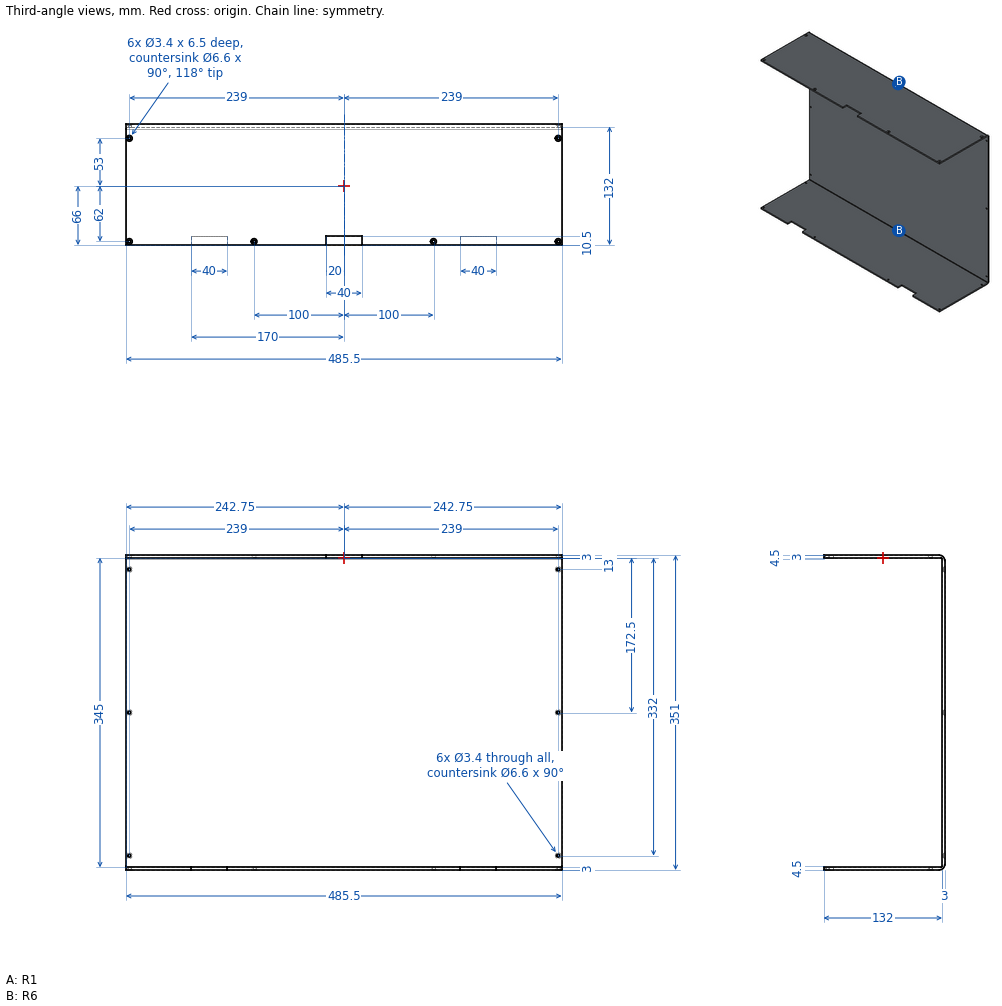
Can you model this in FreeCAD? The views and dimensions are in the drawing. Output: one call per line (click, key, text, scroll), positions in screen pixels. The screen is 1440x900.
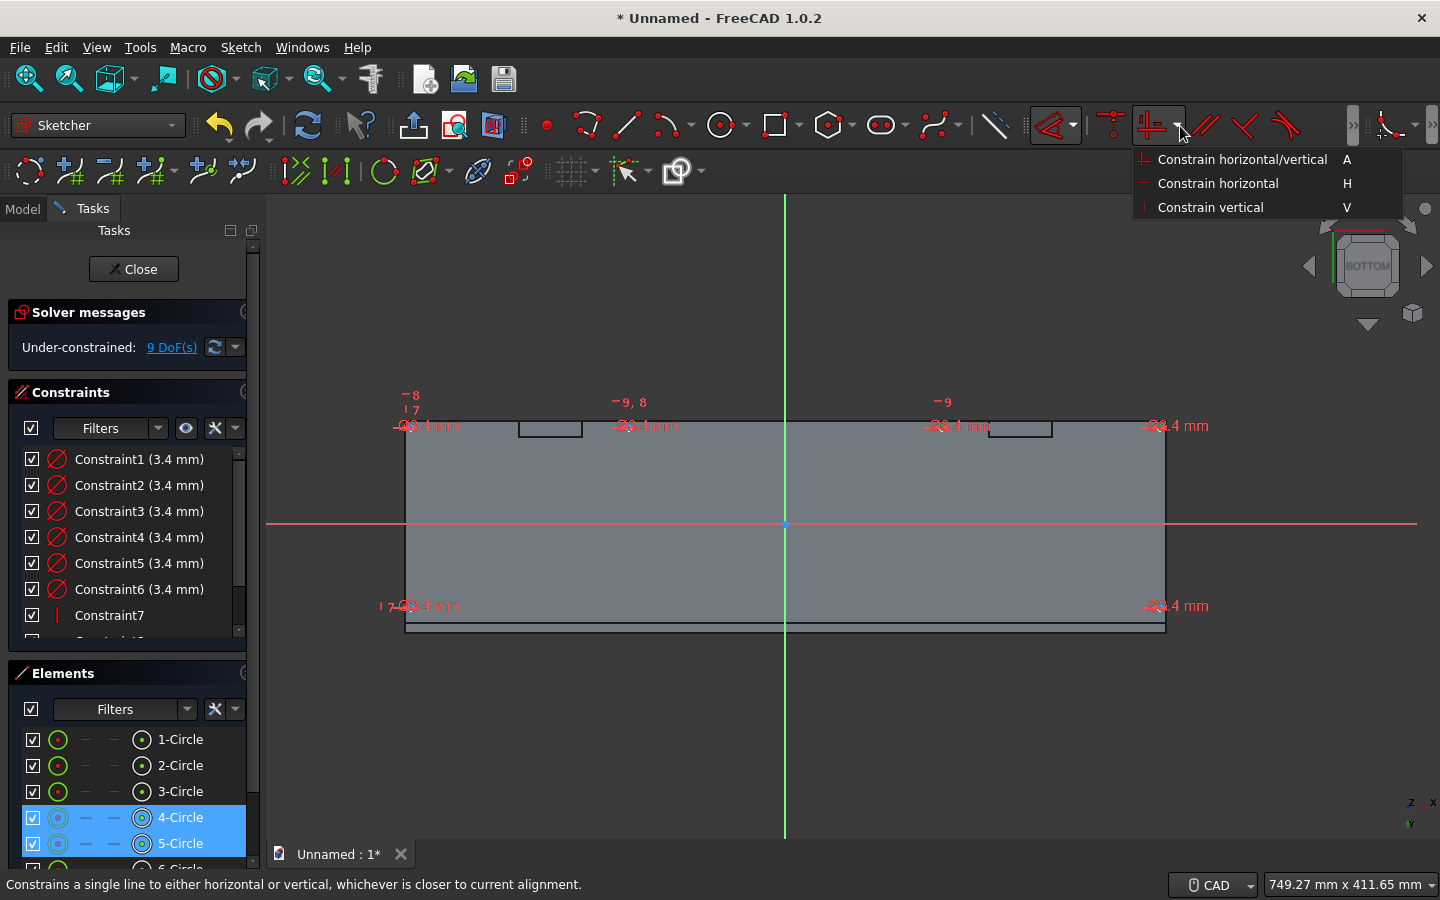
click(1268, 183)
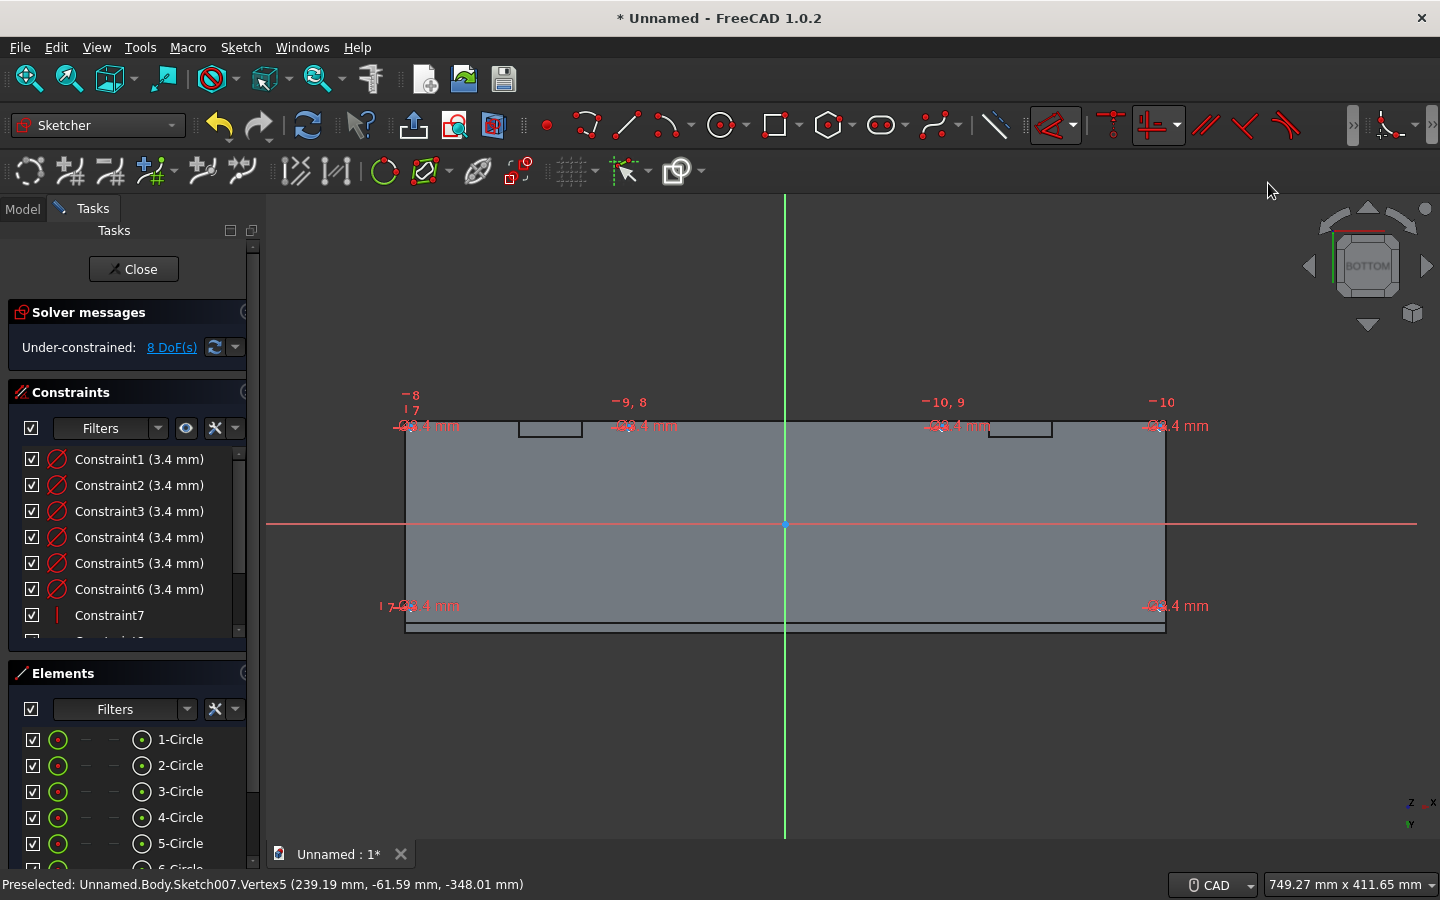
click(1160, 428)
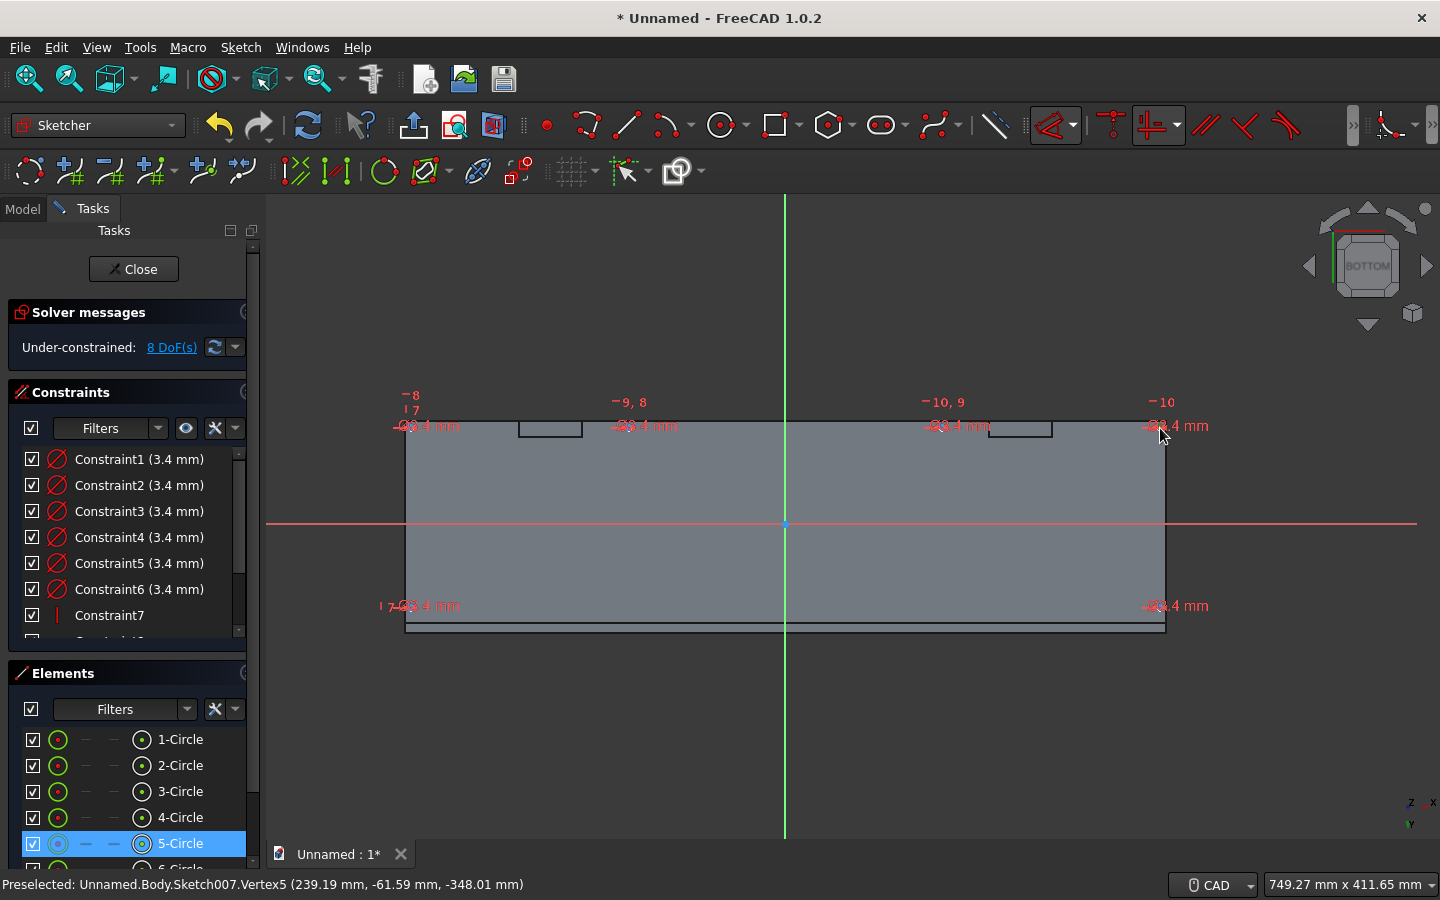
click(1160, 608)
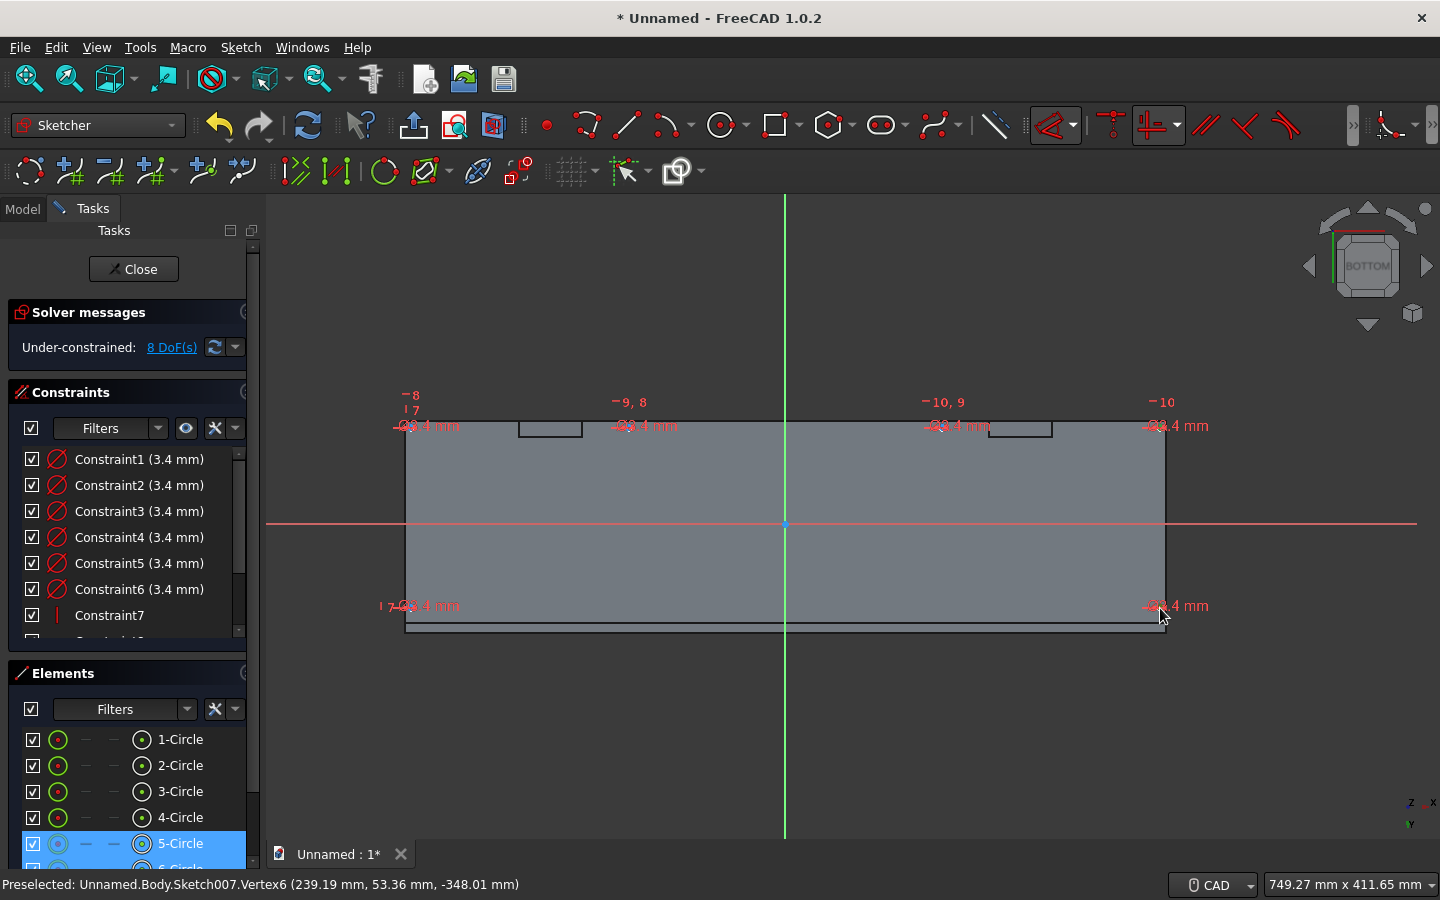
click(1180, 126)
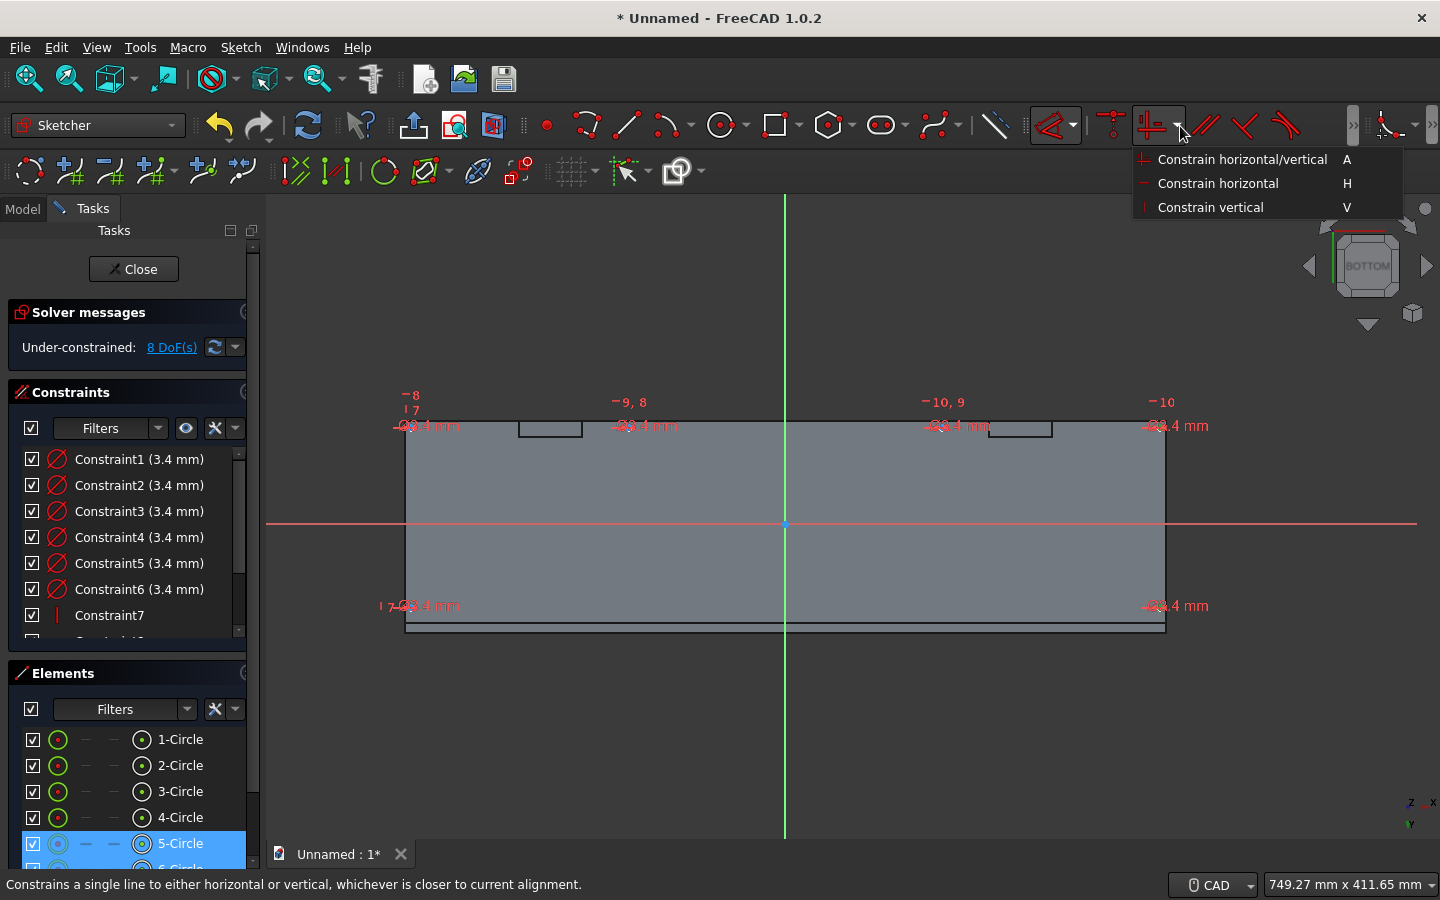
click(1268, 207)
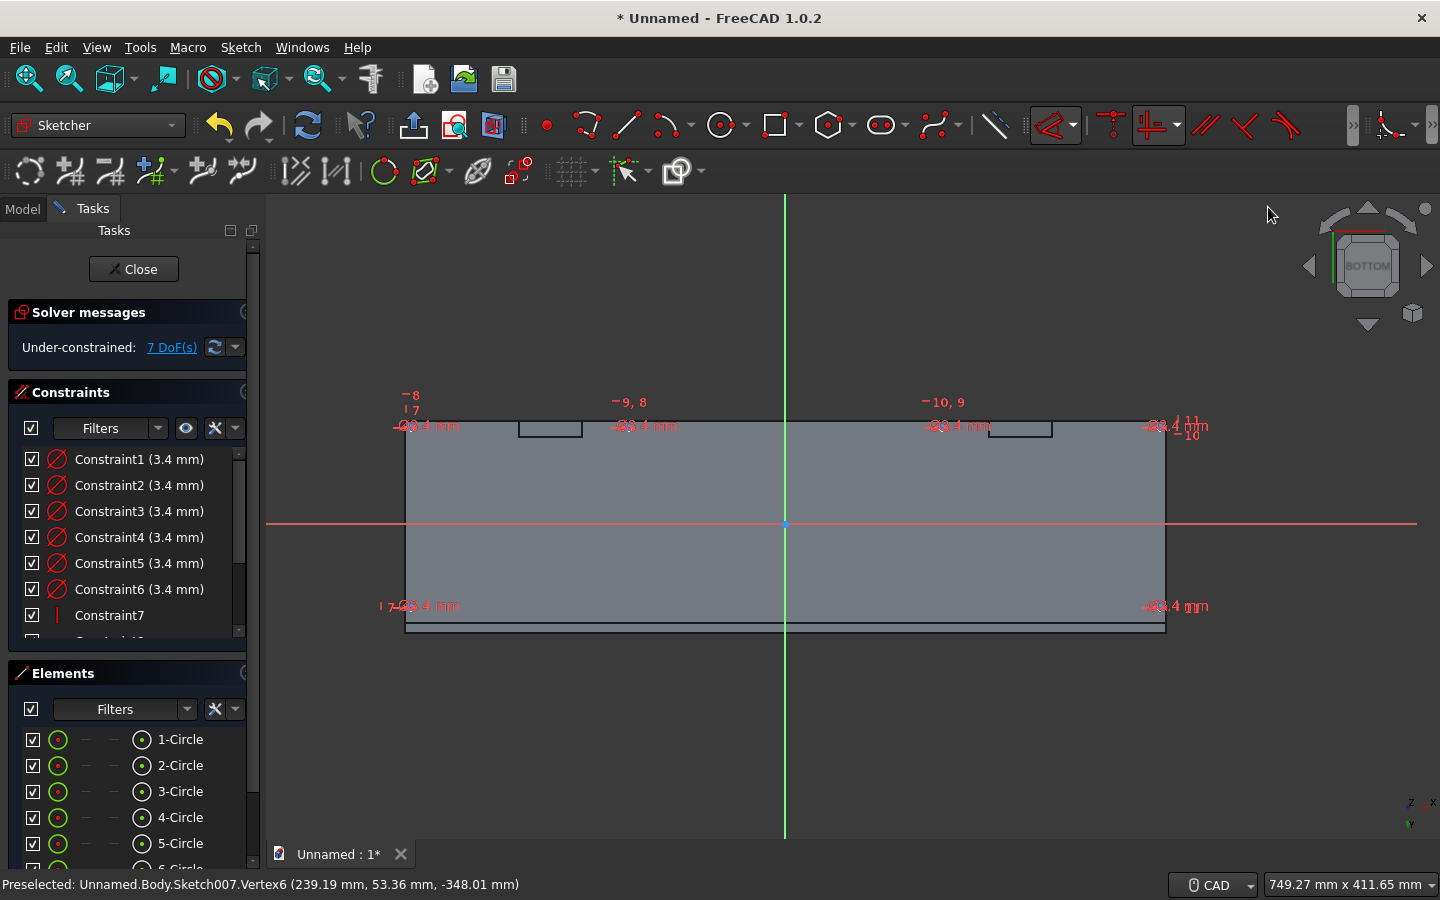
click(411, 608)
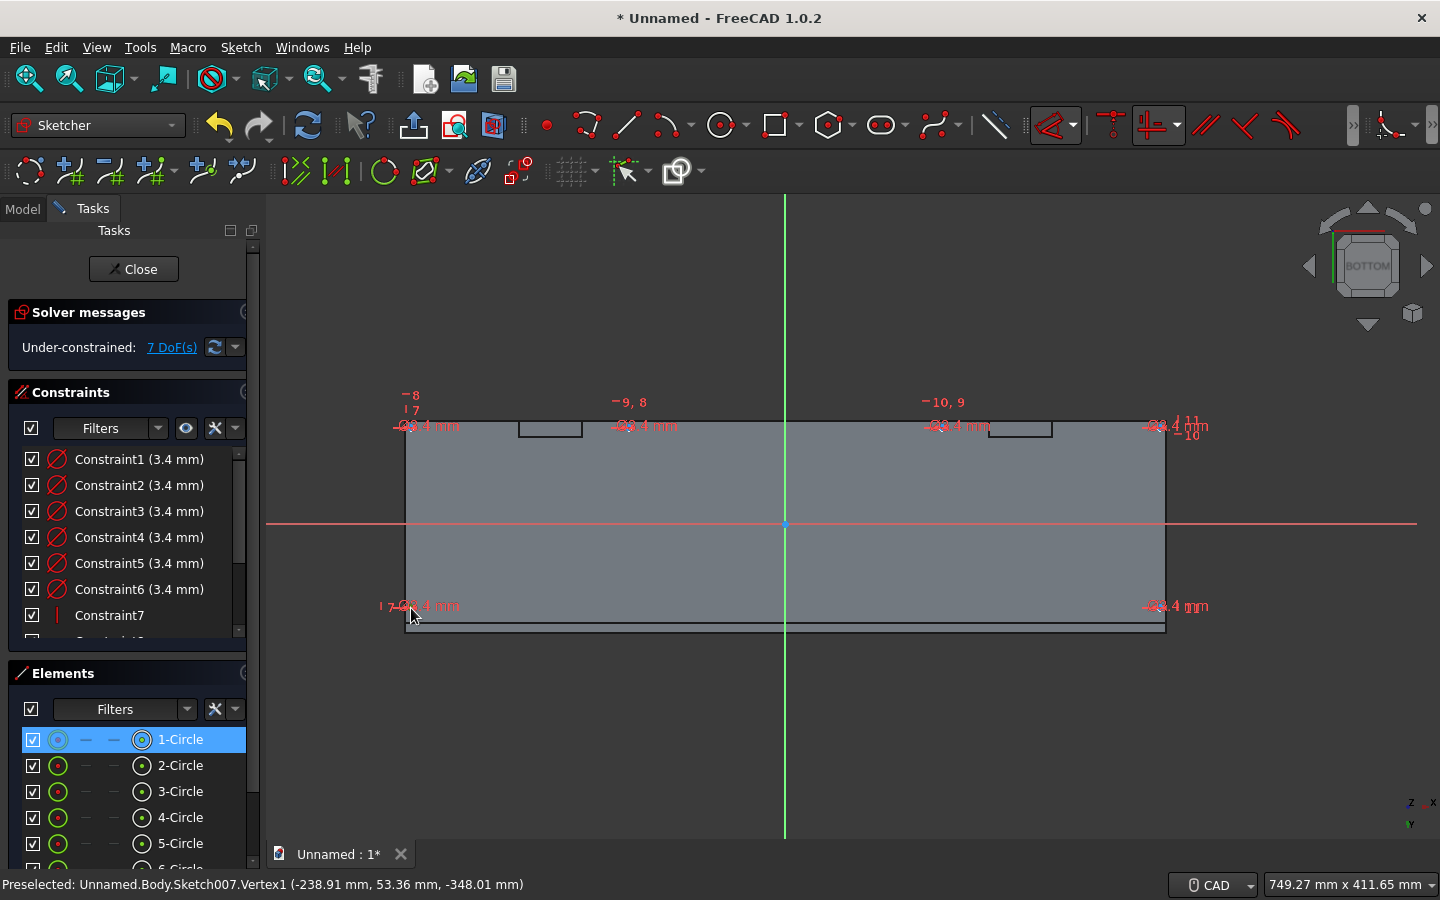
click(1160, 608)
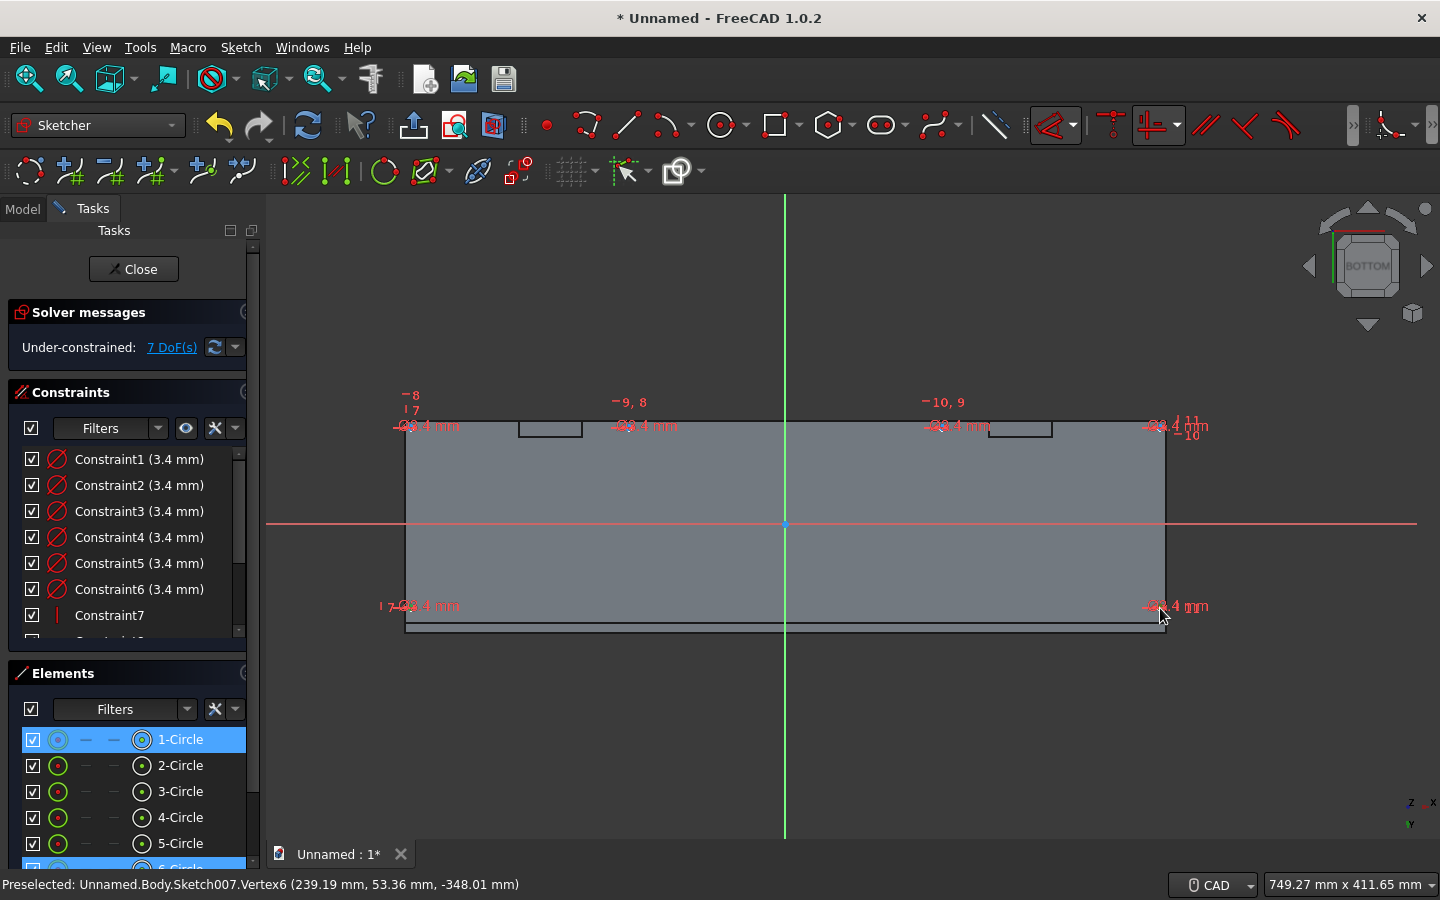
click(1180, 126)